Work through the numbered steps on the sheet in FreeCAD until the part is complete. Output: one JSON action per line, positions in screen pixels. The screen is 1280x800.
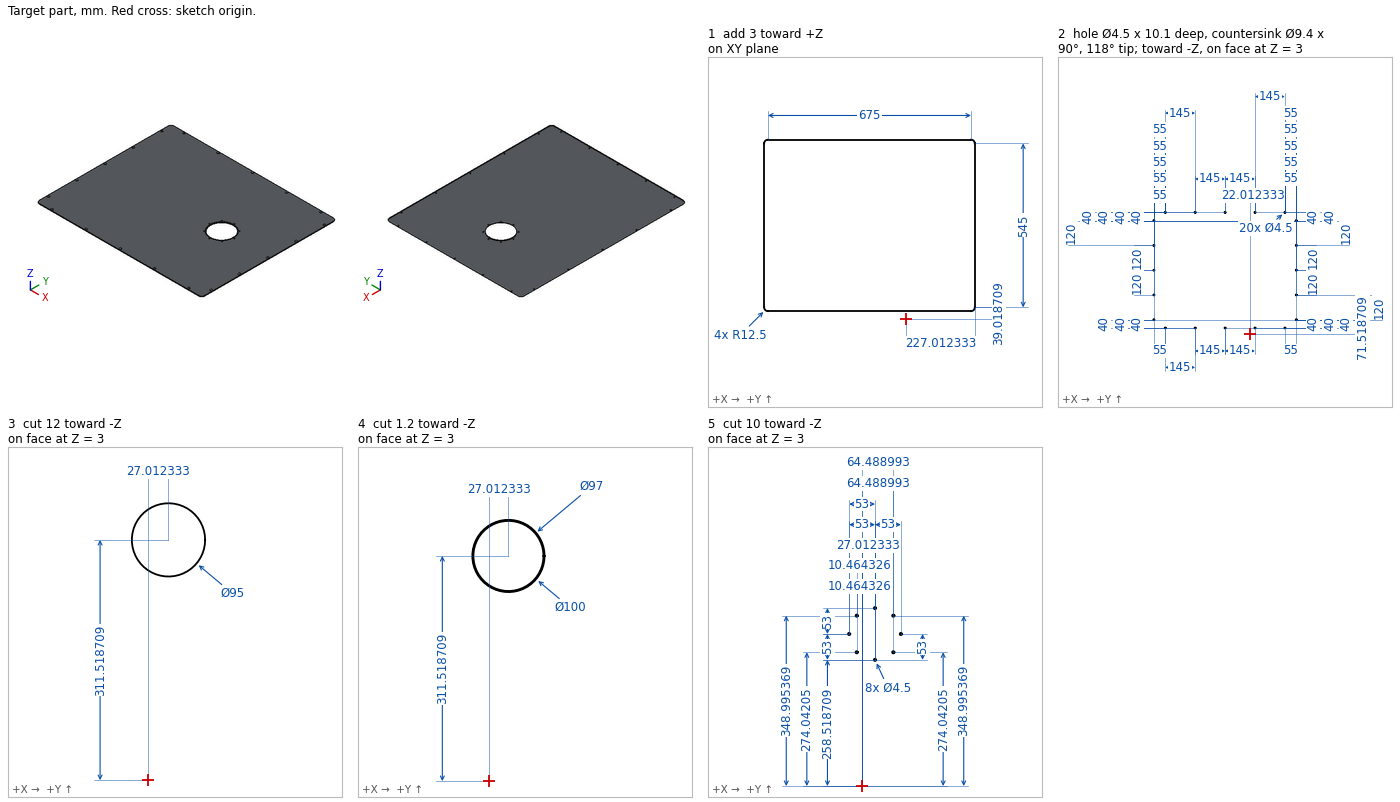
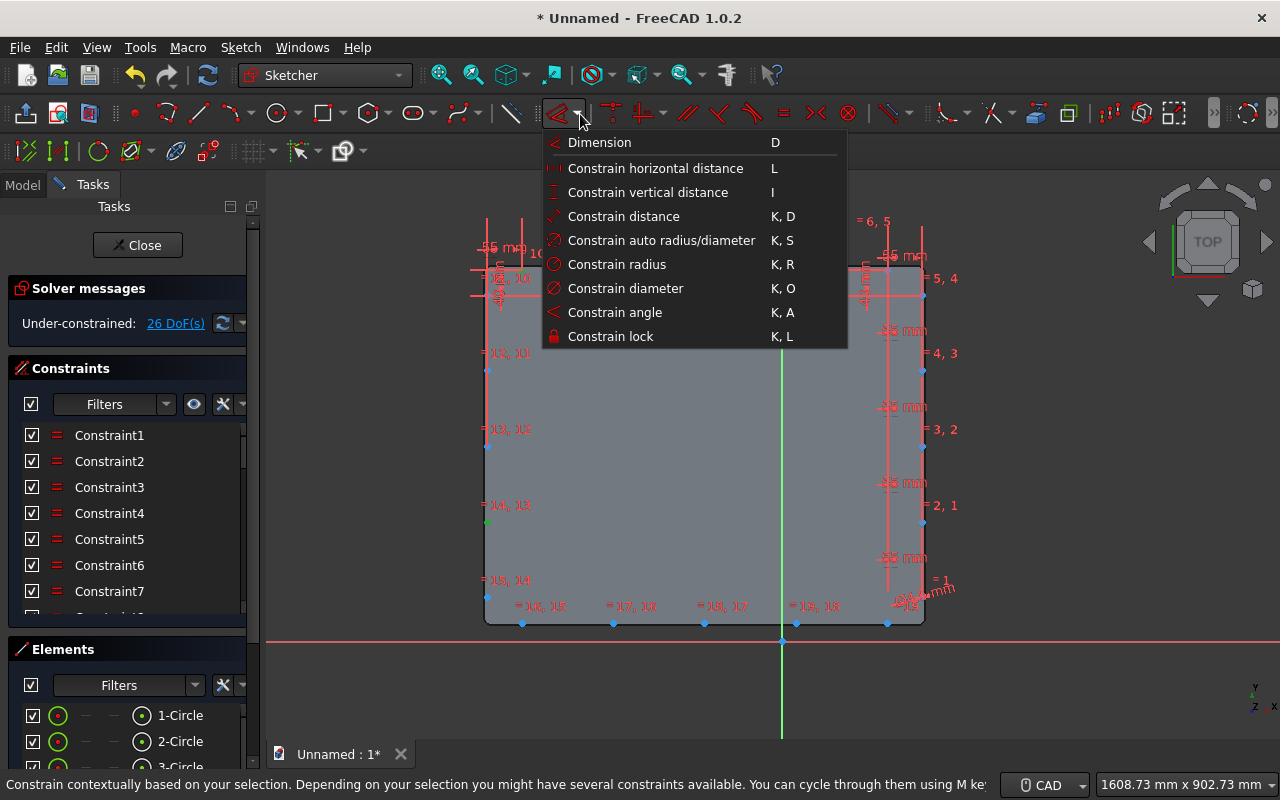
{"action": "left_click", "coordinate": [695, 168]}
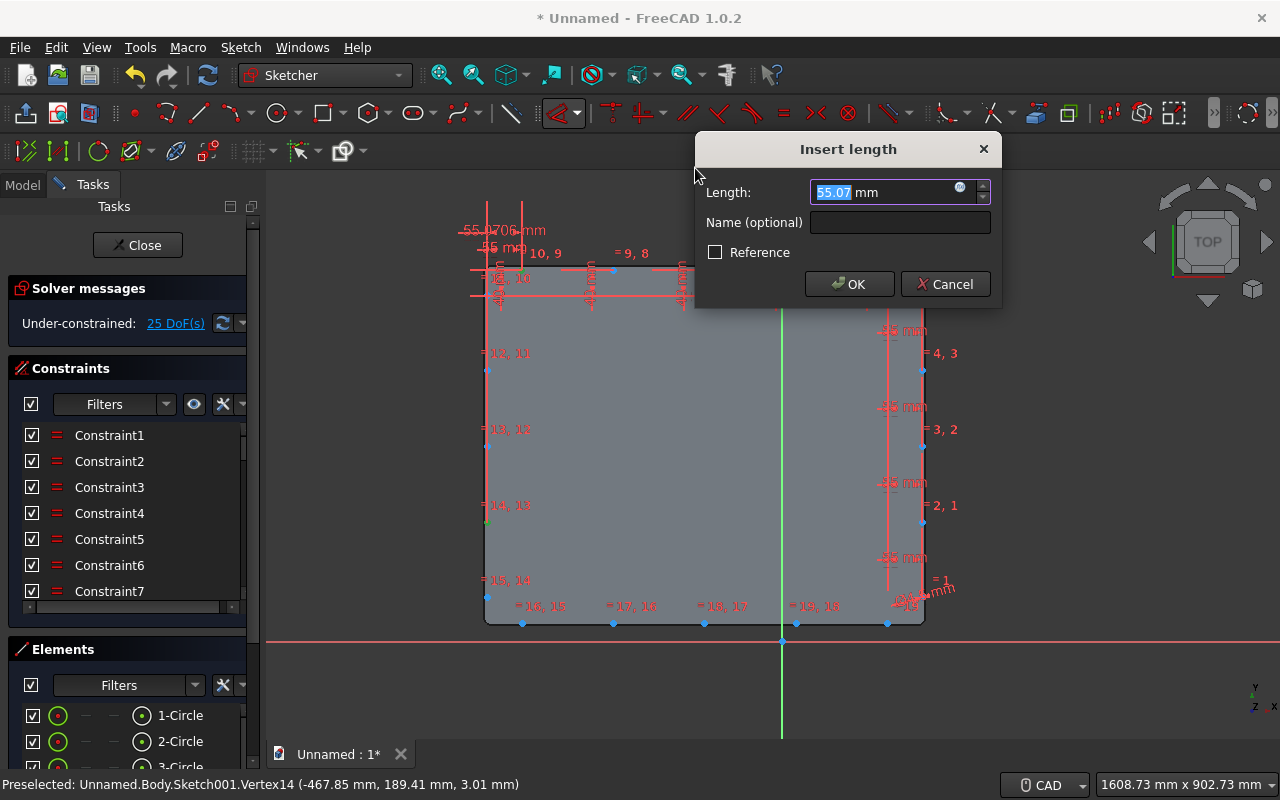
{"action": "type", "text": "55"}
{"action": "key", "text": "Return"}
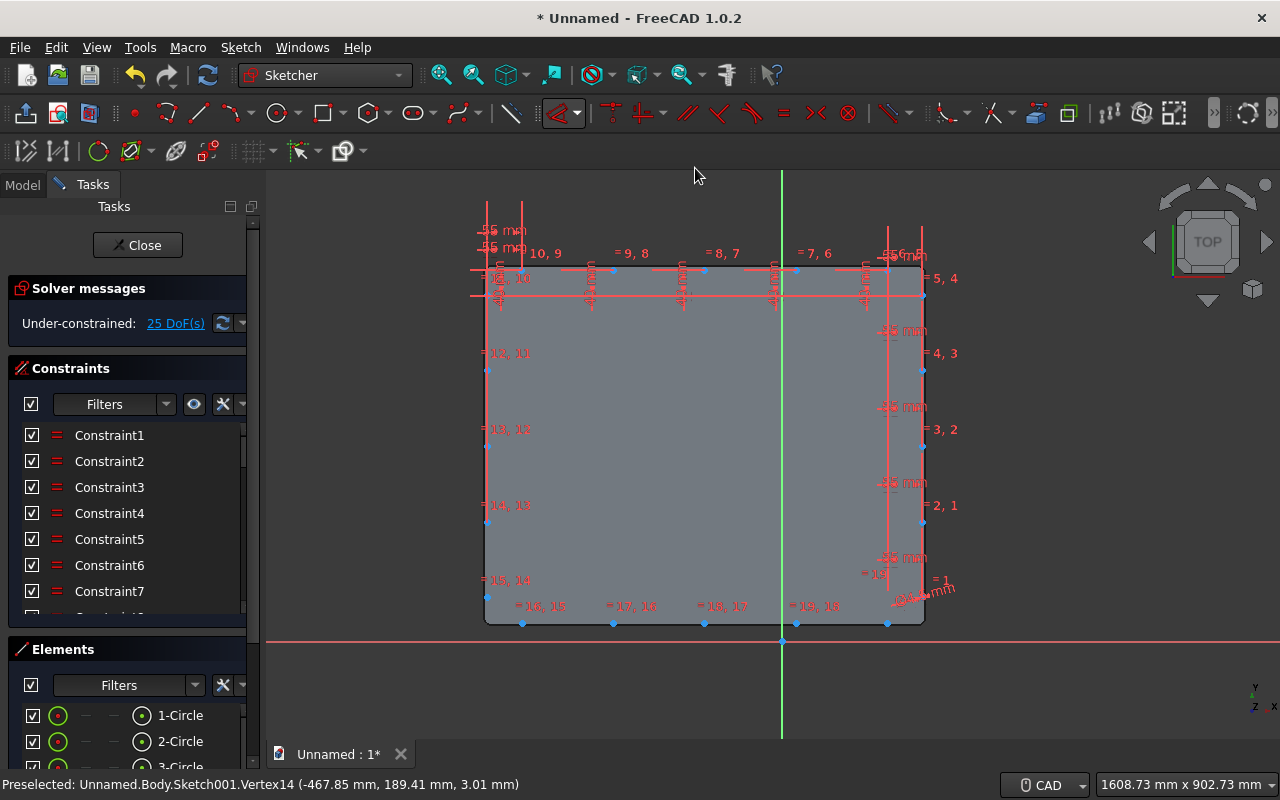
{"action": "left_click", "coordinate": [522, 270]}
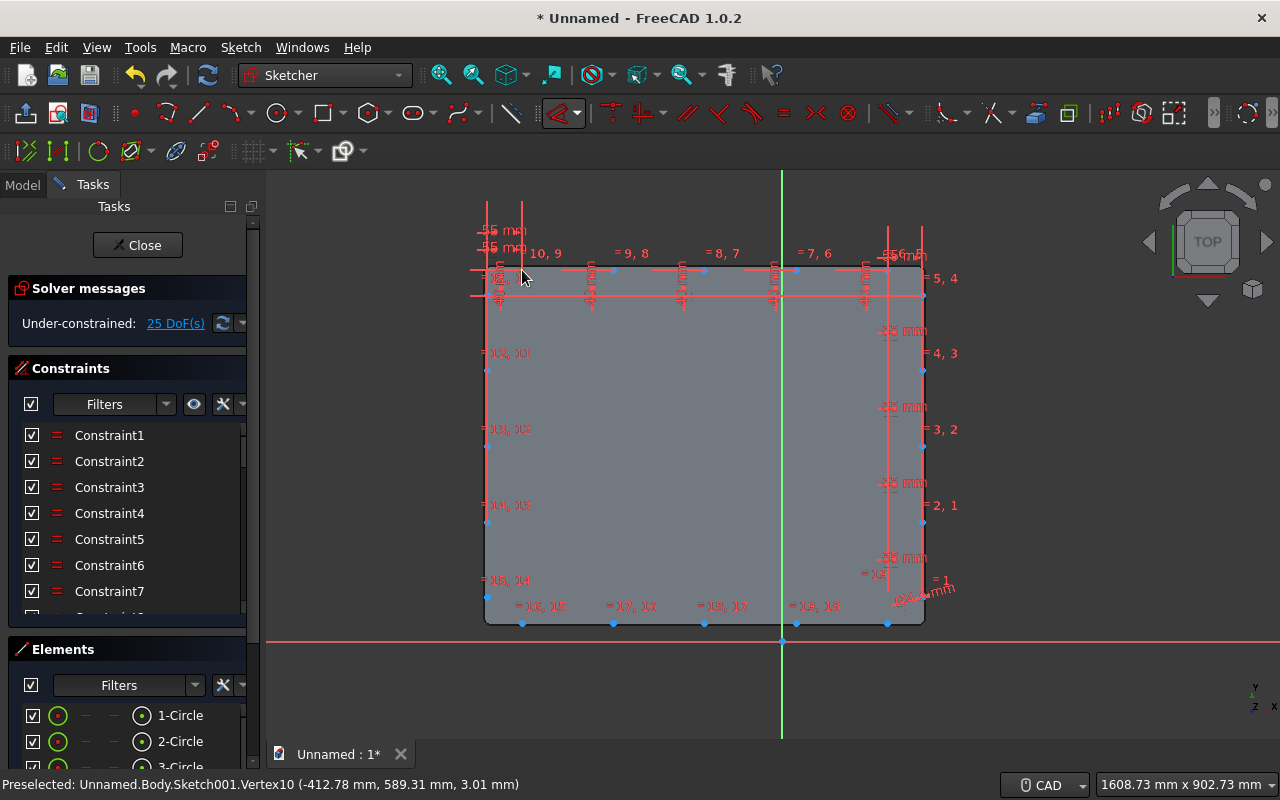
{"action": "left_click", "coordinate": [487, 597]}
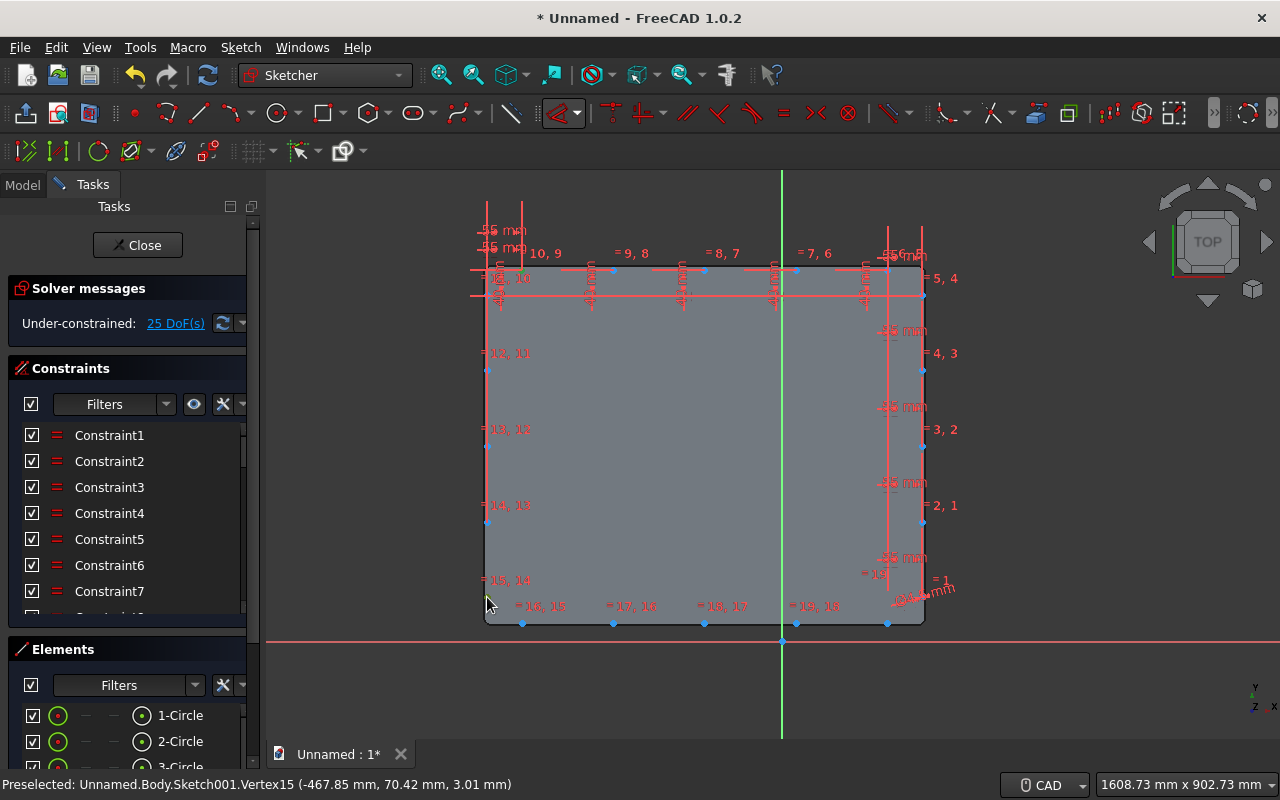
{"action": "key", "text": "l"}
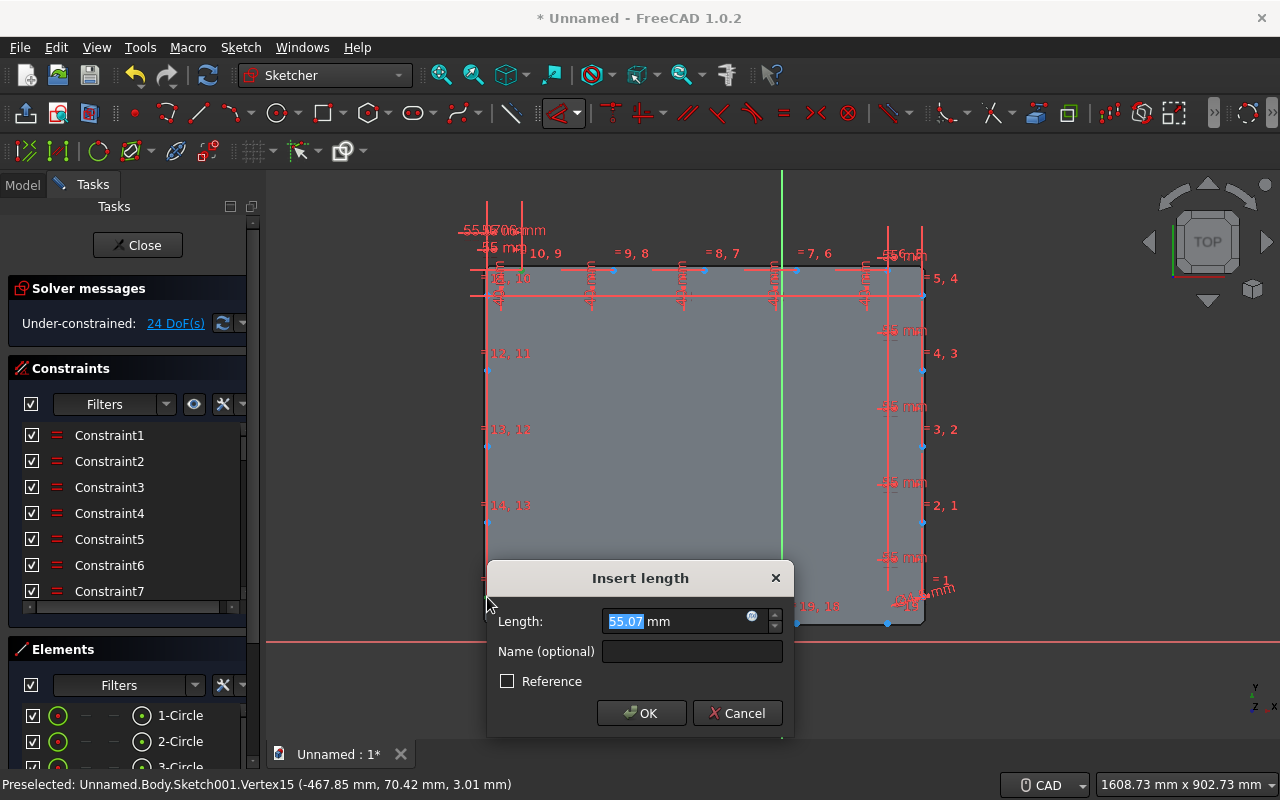
{"action": "type", "text": "55"}
{"action": "key", "text": "Return"}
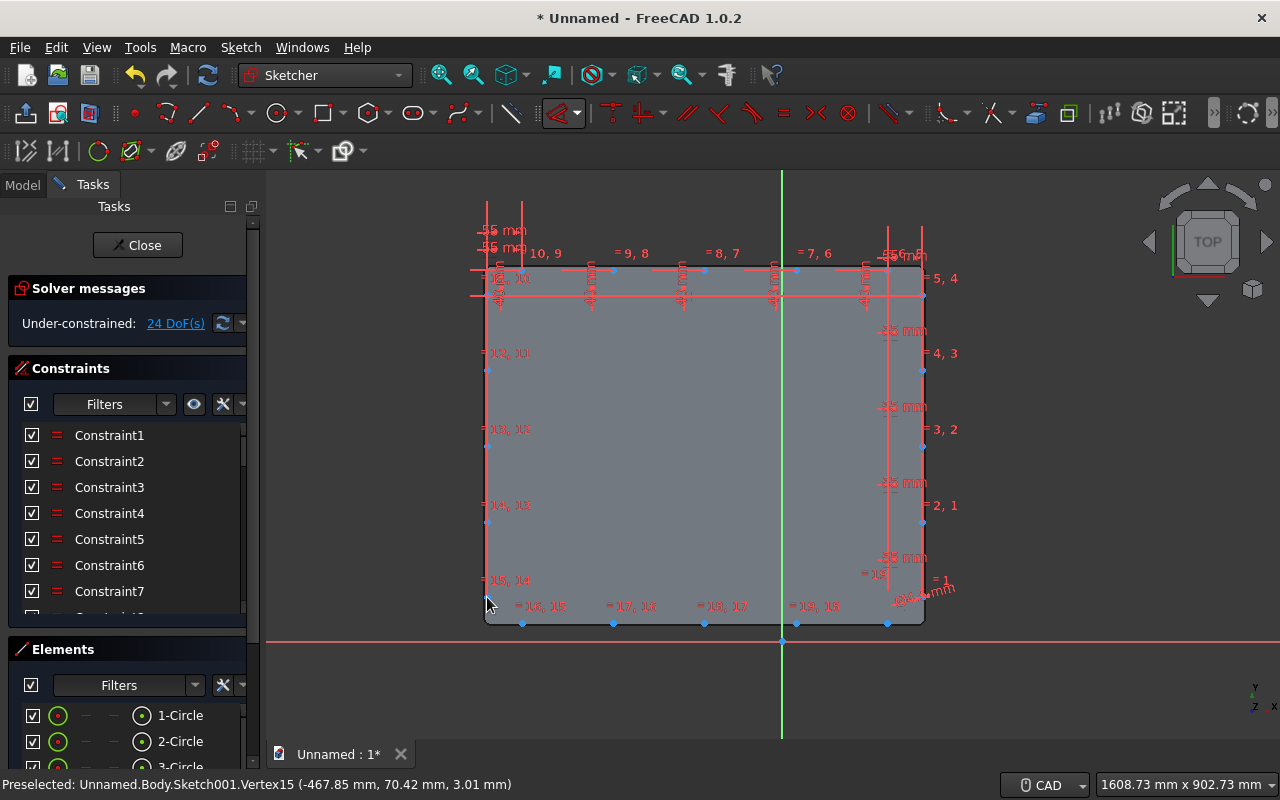
{"action": "left_click", "coordinate": [487, 597]}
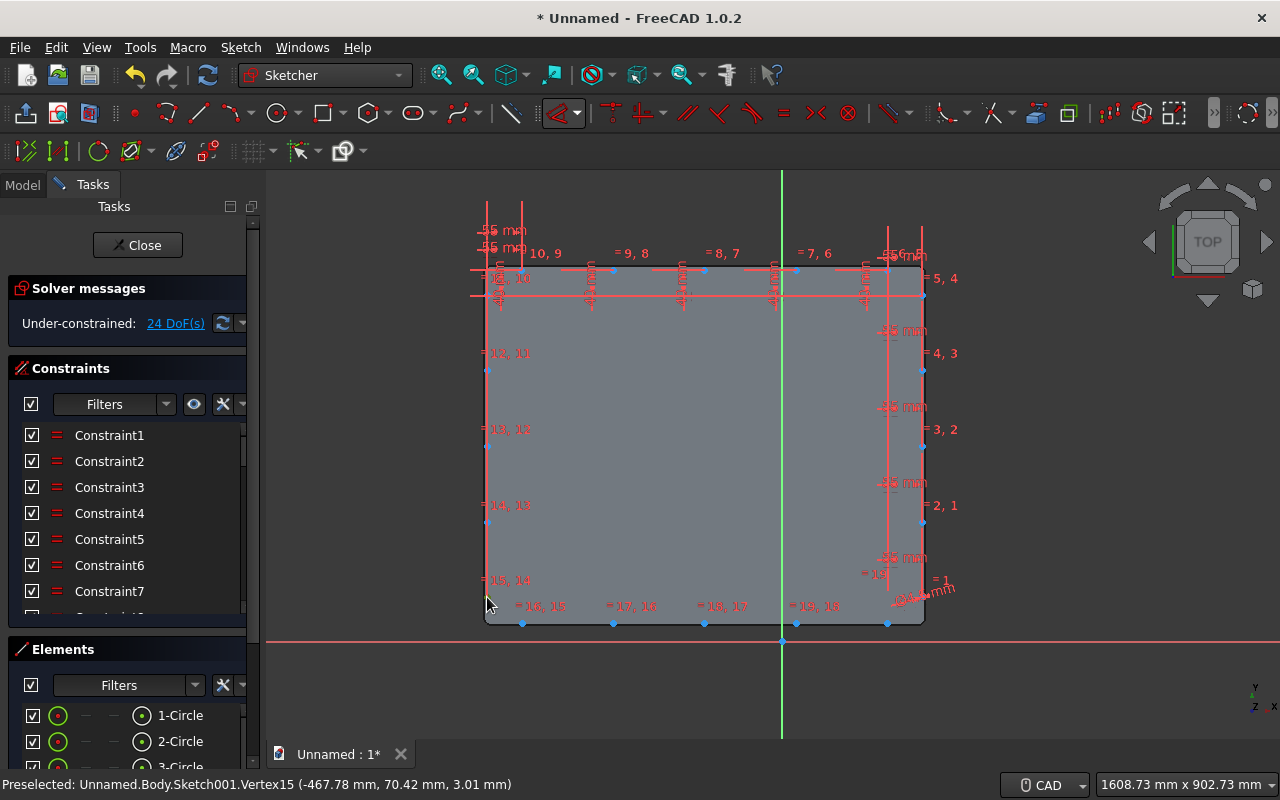
{"action": "left_click", "coordinate": [522, 623]}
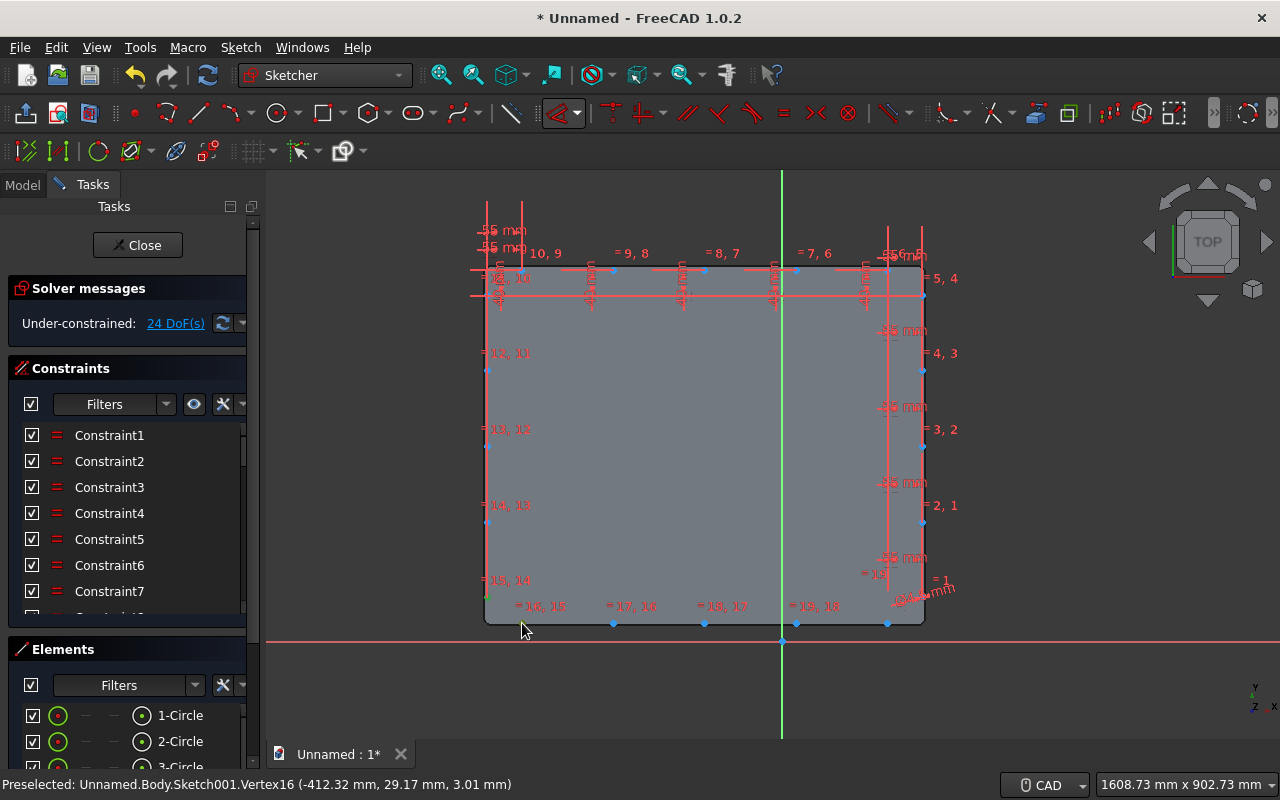
{"action": "left_click", "coordinate": [580, 114]}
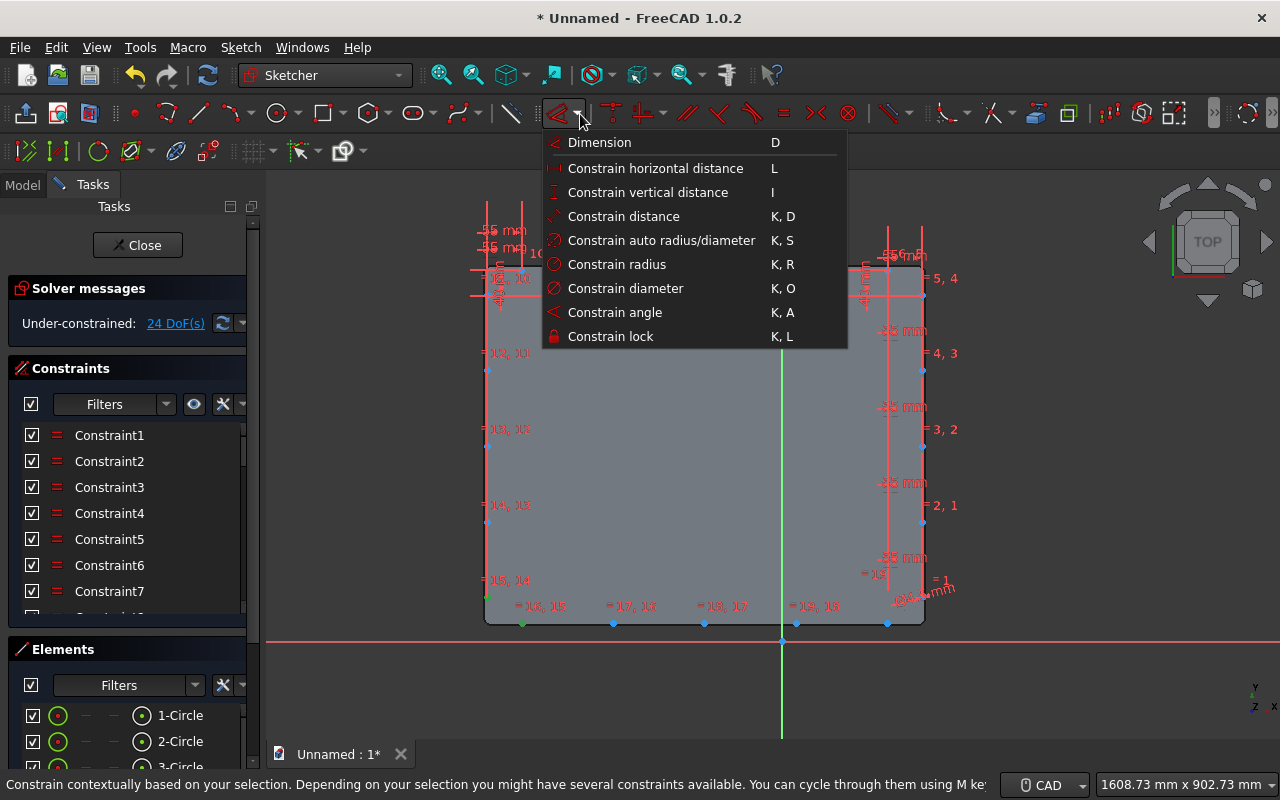
{"action": "left_click", "coordinate": [695, 168]}